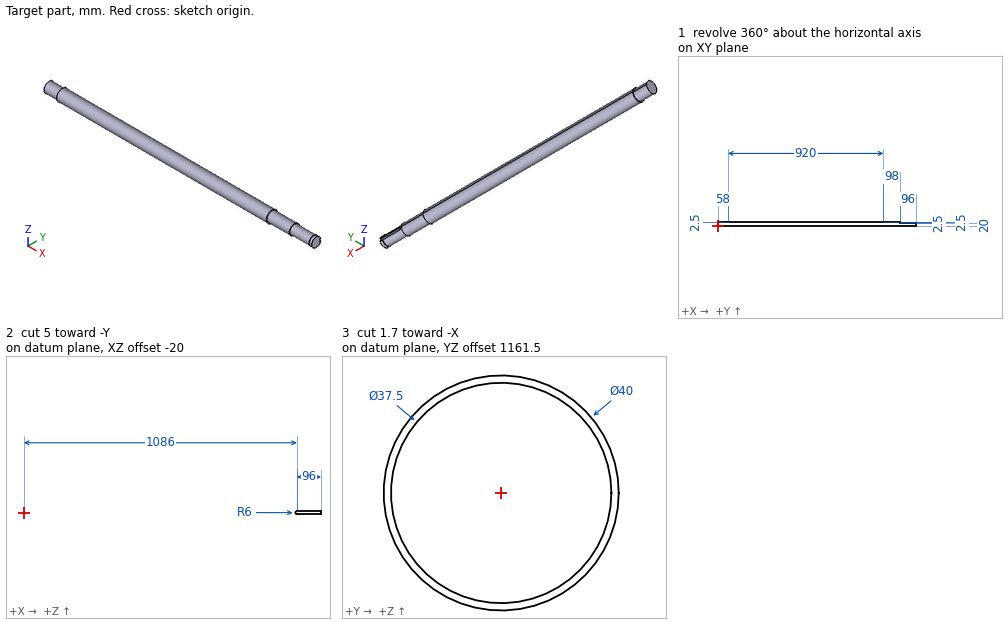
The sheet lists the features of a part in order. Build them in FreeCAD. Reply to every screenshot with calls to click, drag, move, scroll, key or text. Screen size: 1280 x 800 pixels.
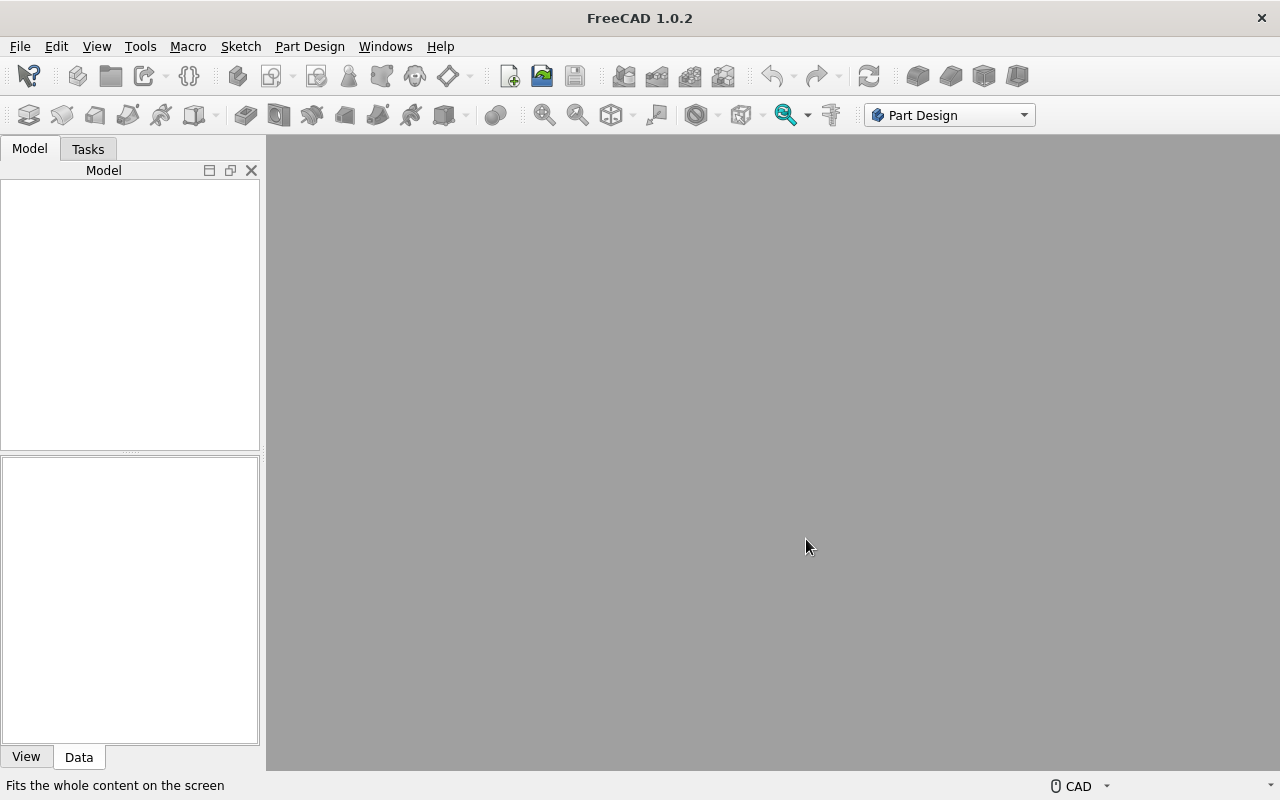
click(509, 76)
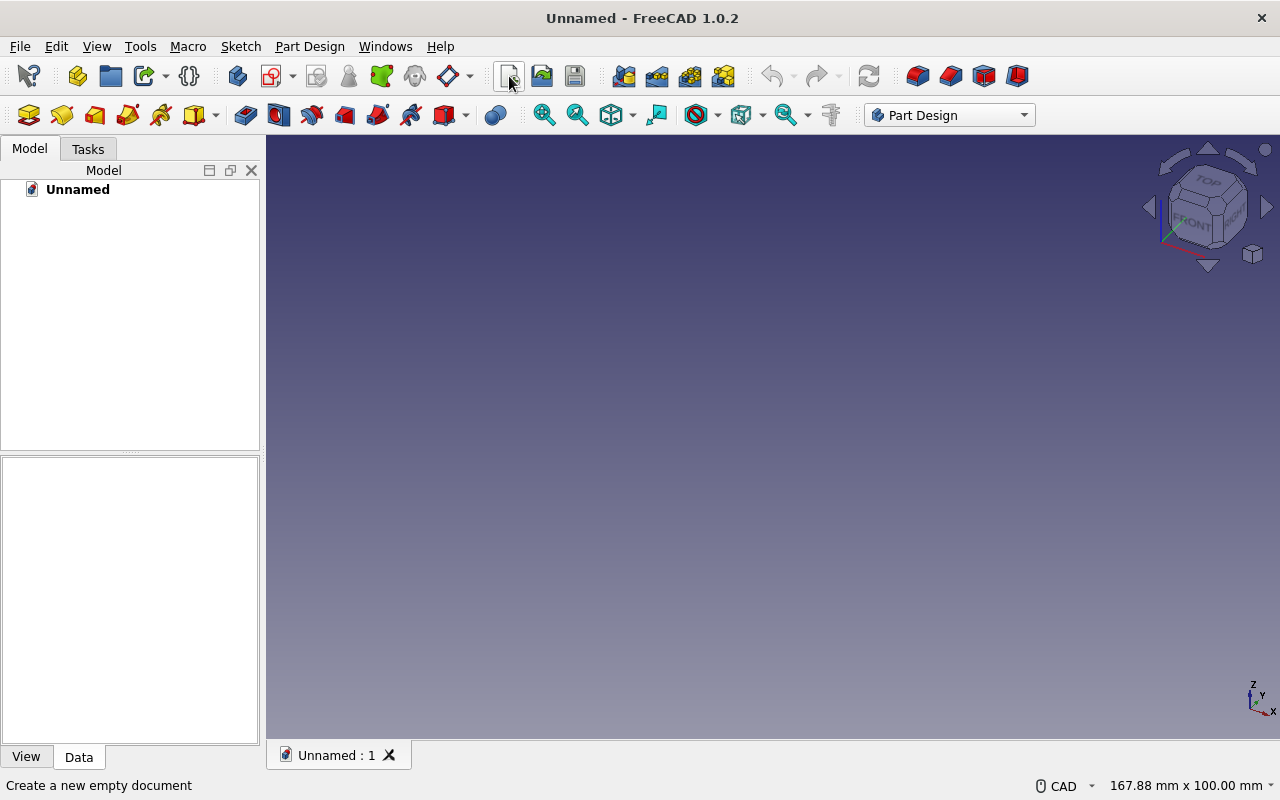
click(270, 76)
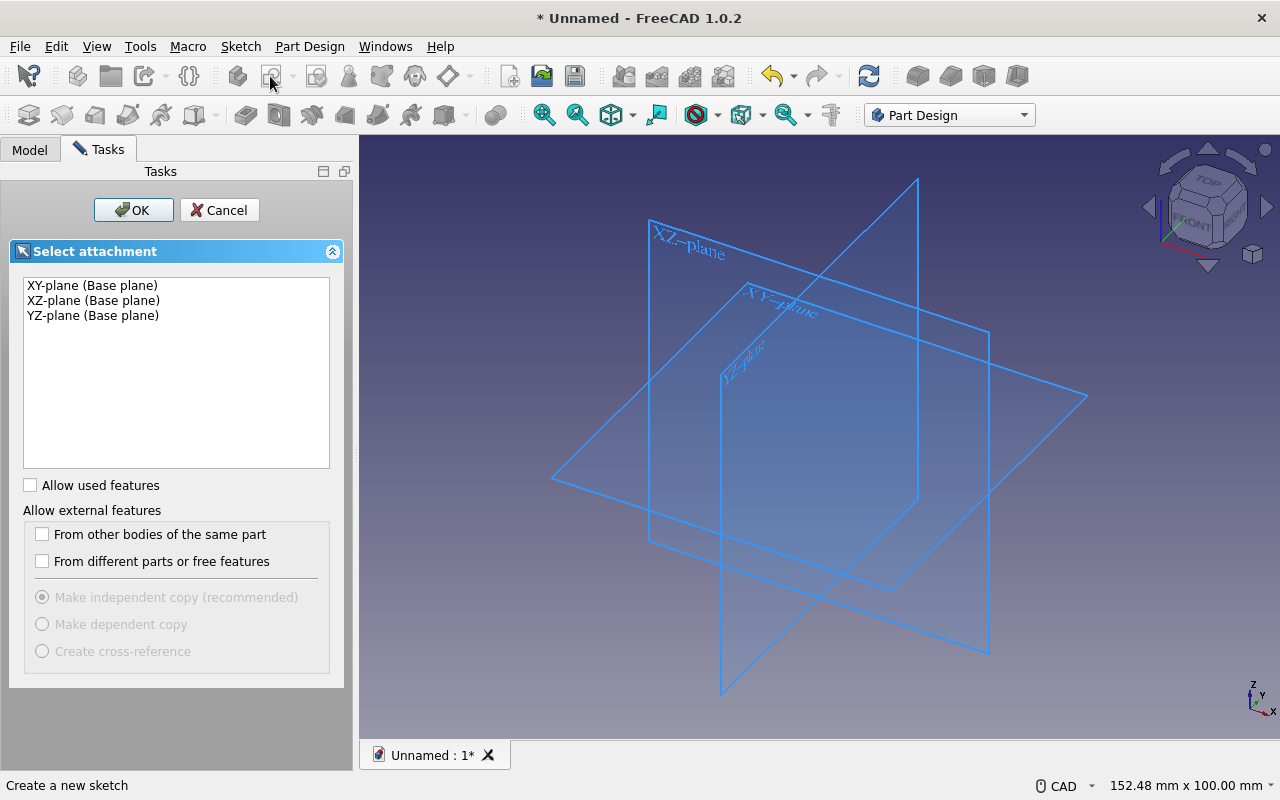
click(84, 286)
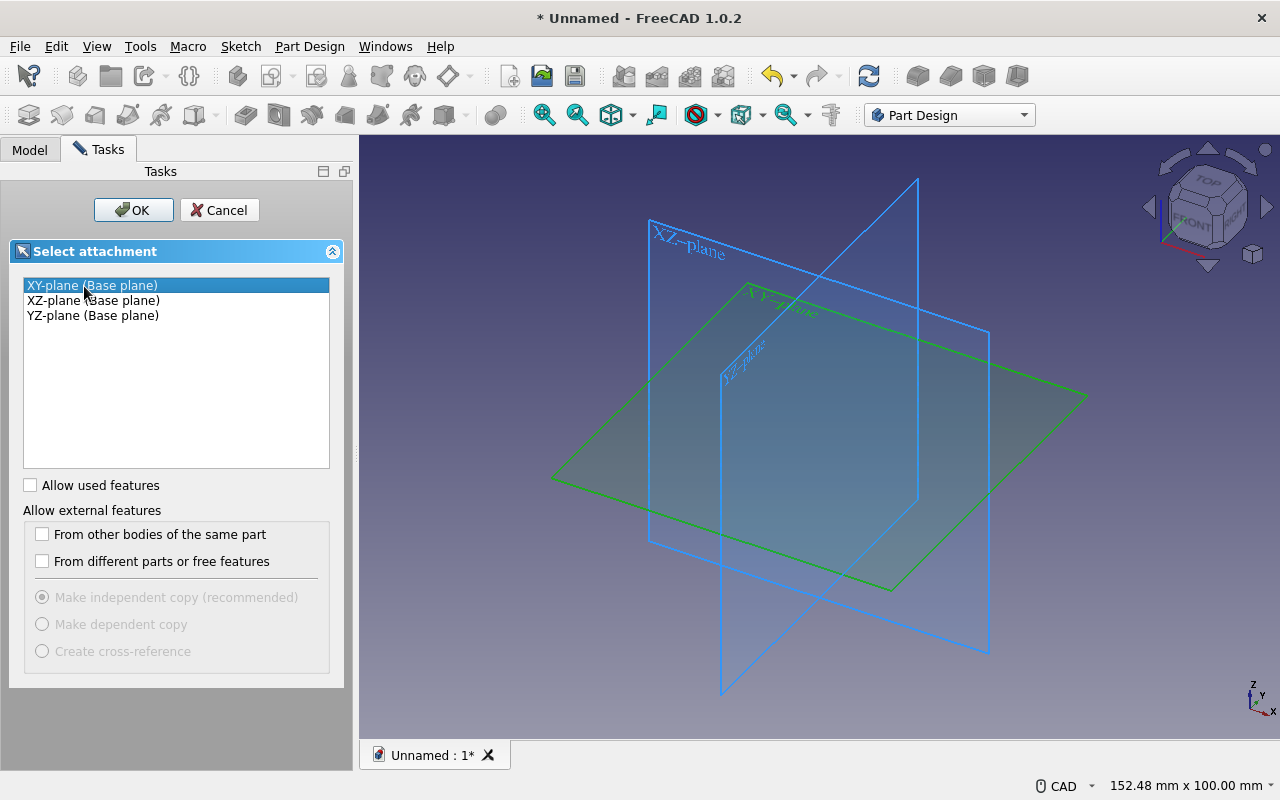
click(134, 210)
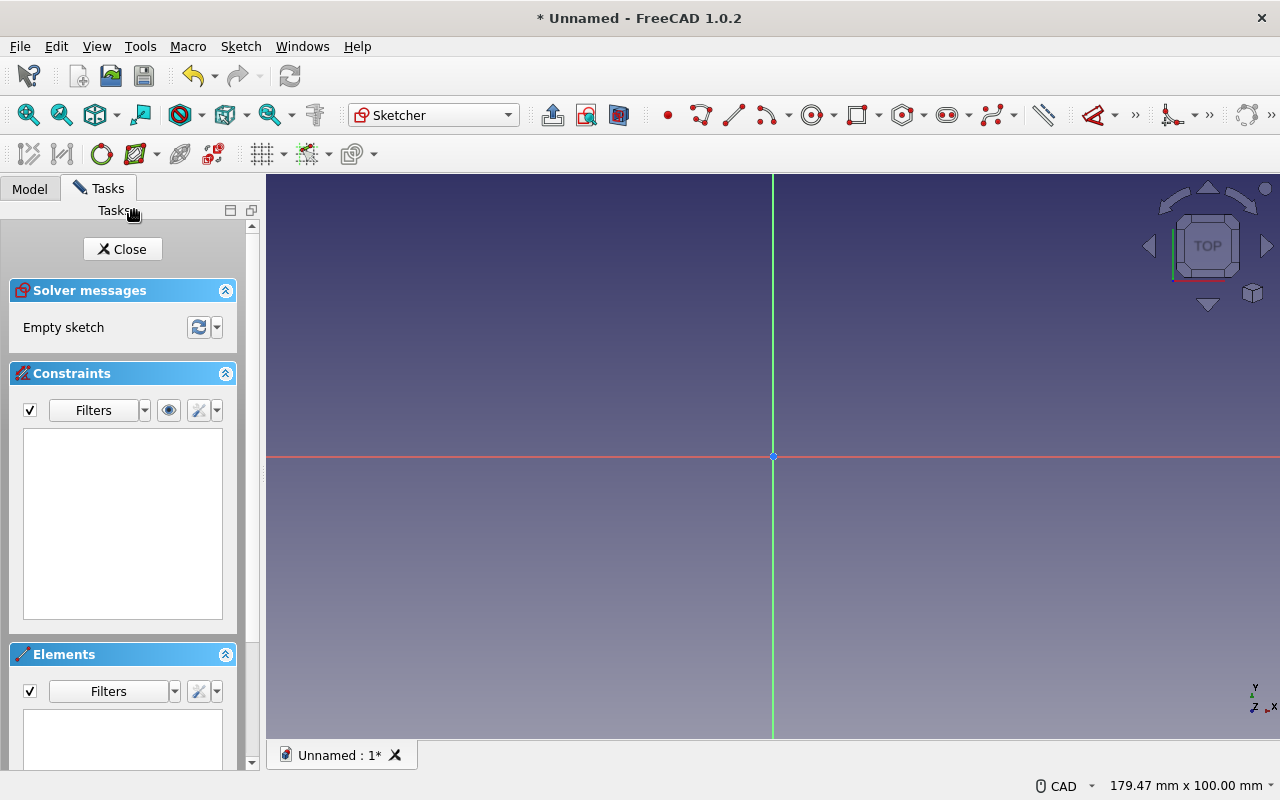
scroll(367, 464, down, 12)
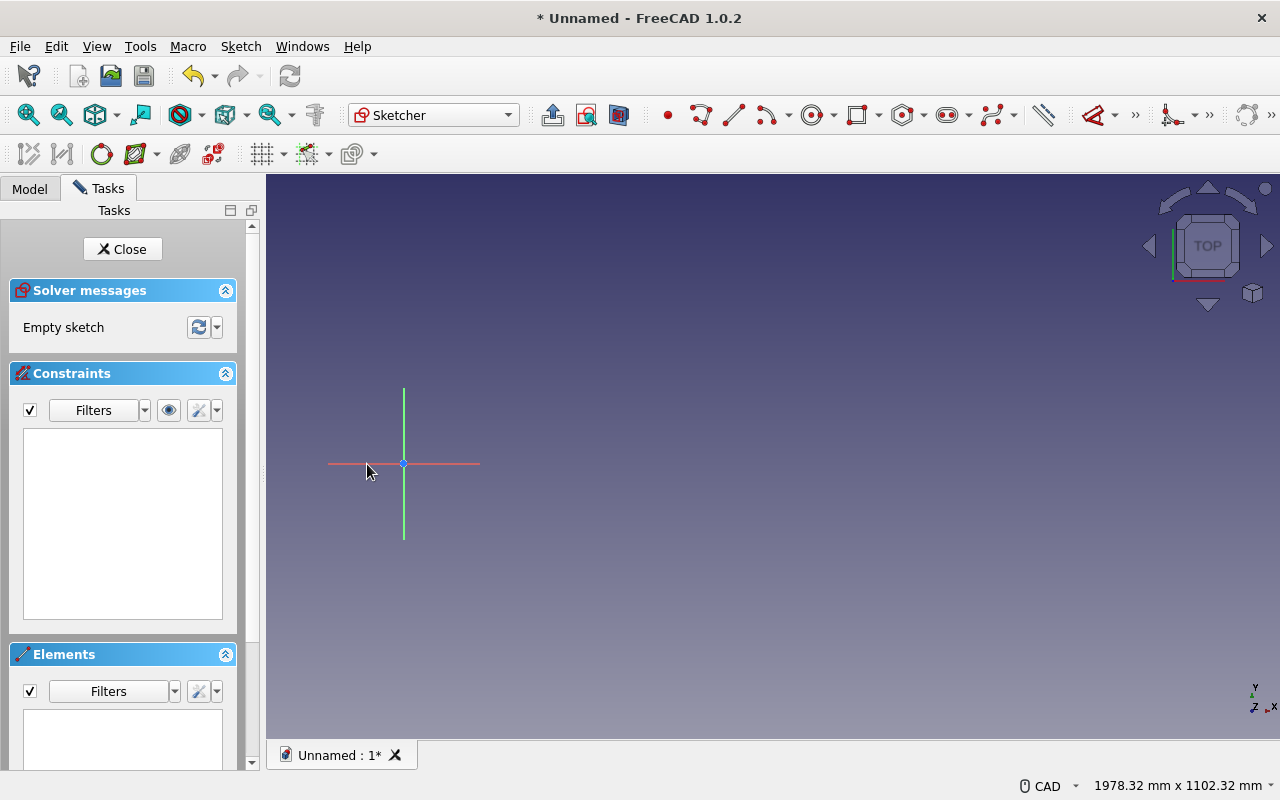
click(701, 116)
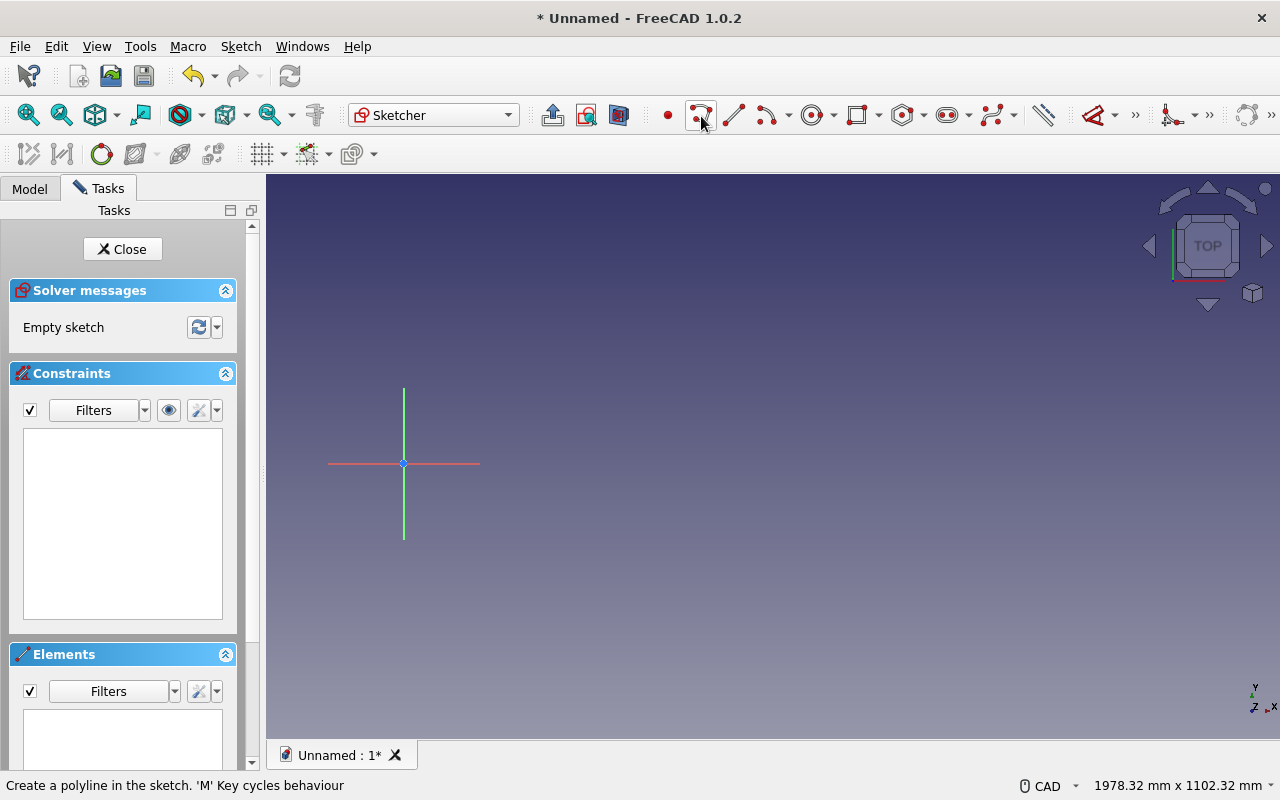
click(404, 464)
click(1005, 455)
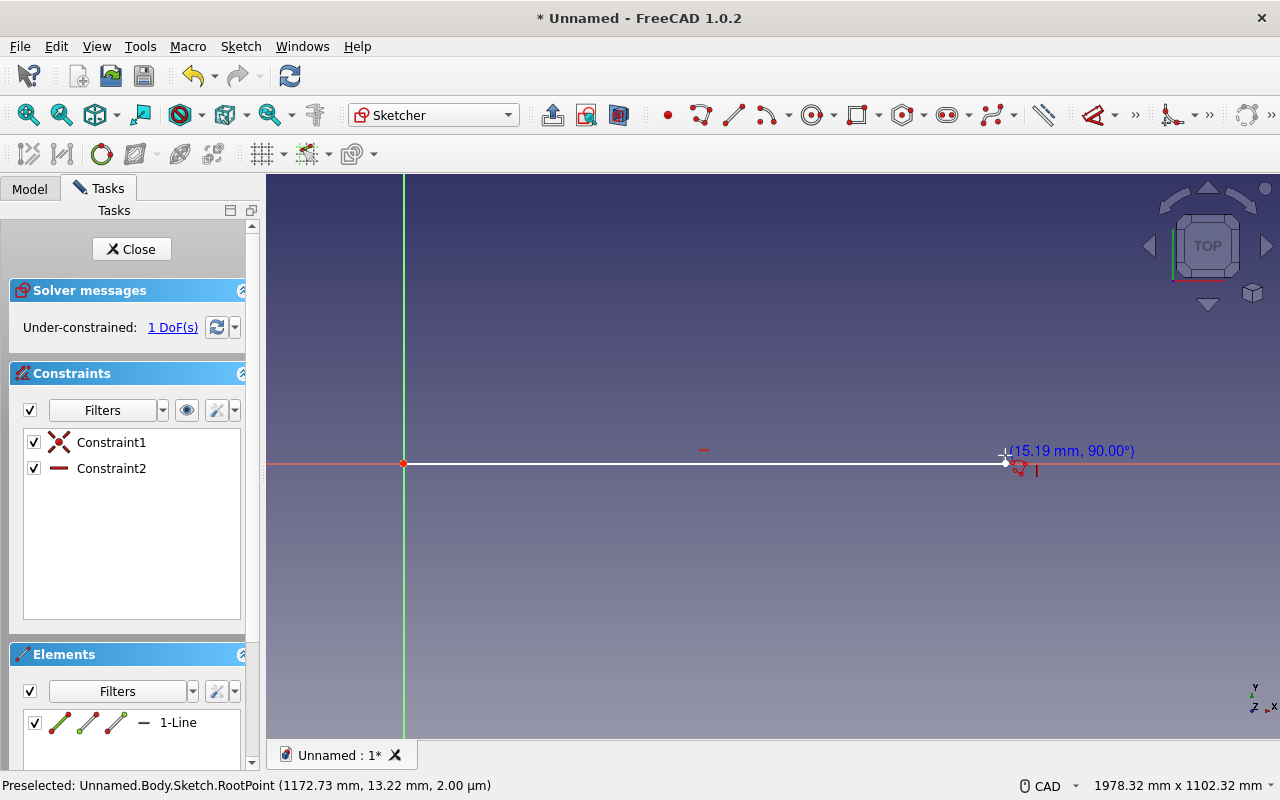
scroll(1005, 454, up, 3)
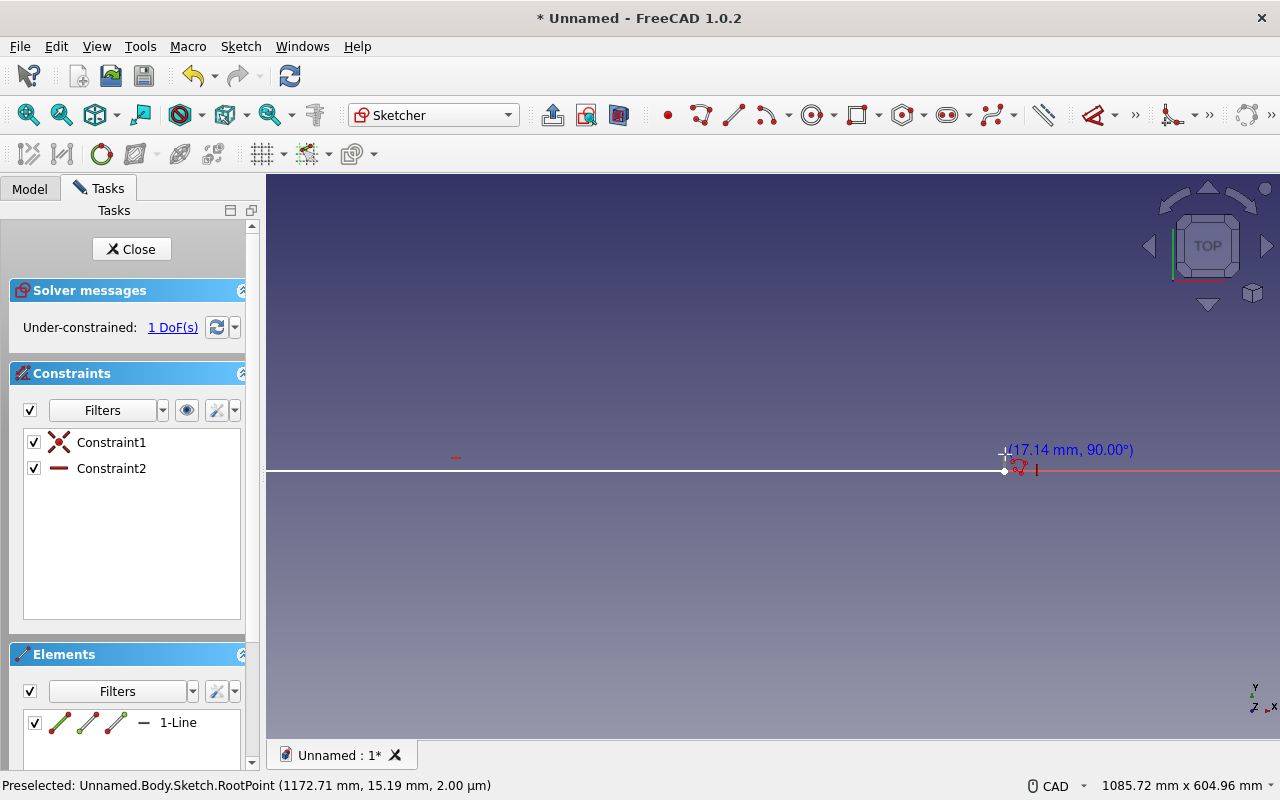
click(1004, 453)
click(914, 453)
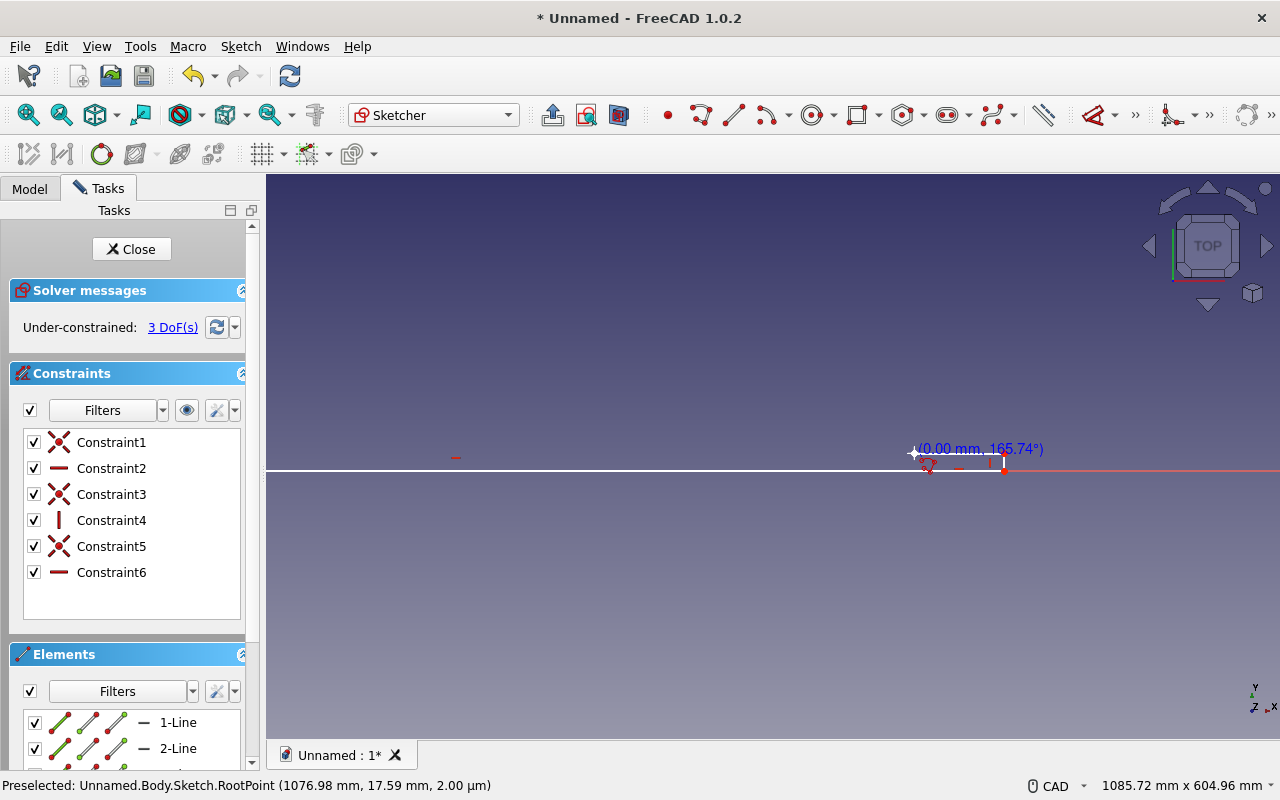
scroll(914, 450, up, 10)